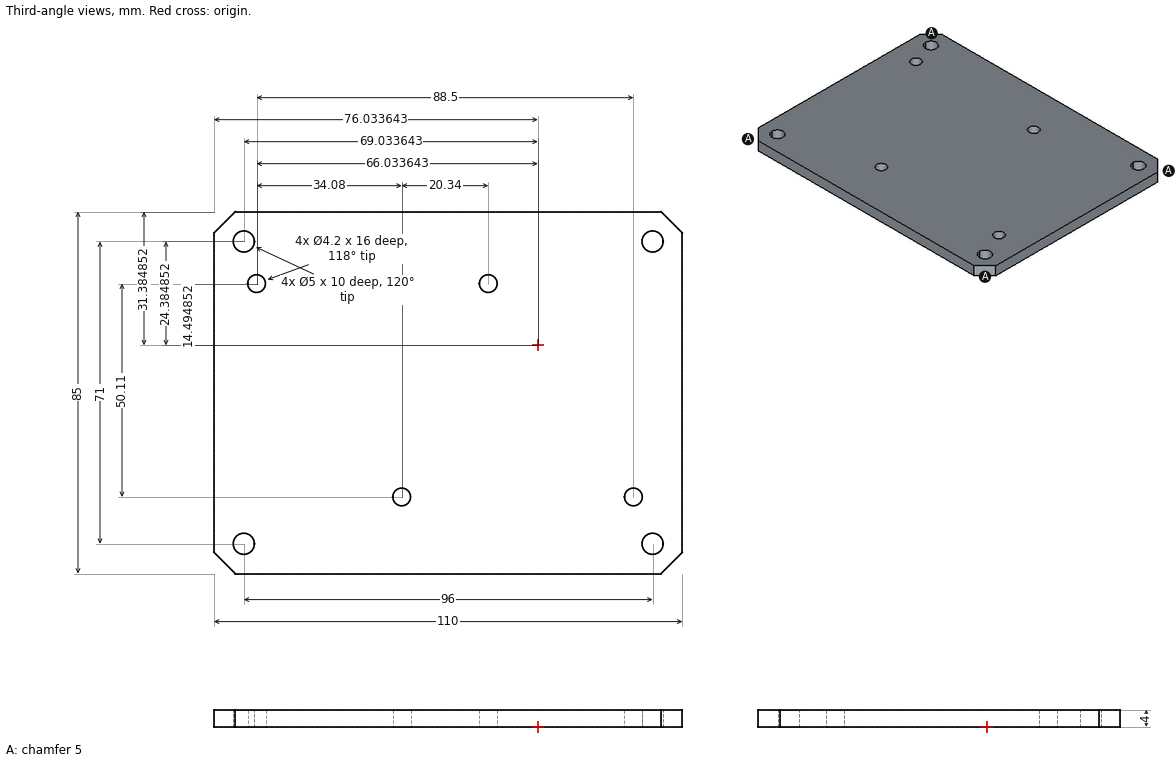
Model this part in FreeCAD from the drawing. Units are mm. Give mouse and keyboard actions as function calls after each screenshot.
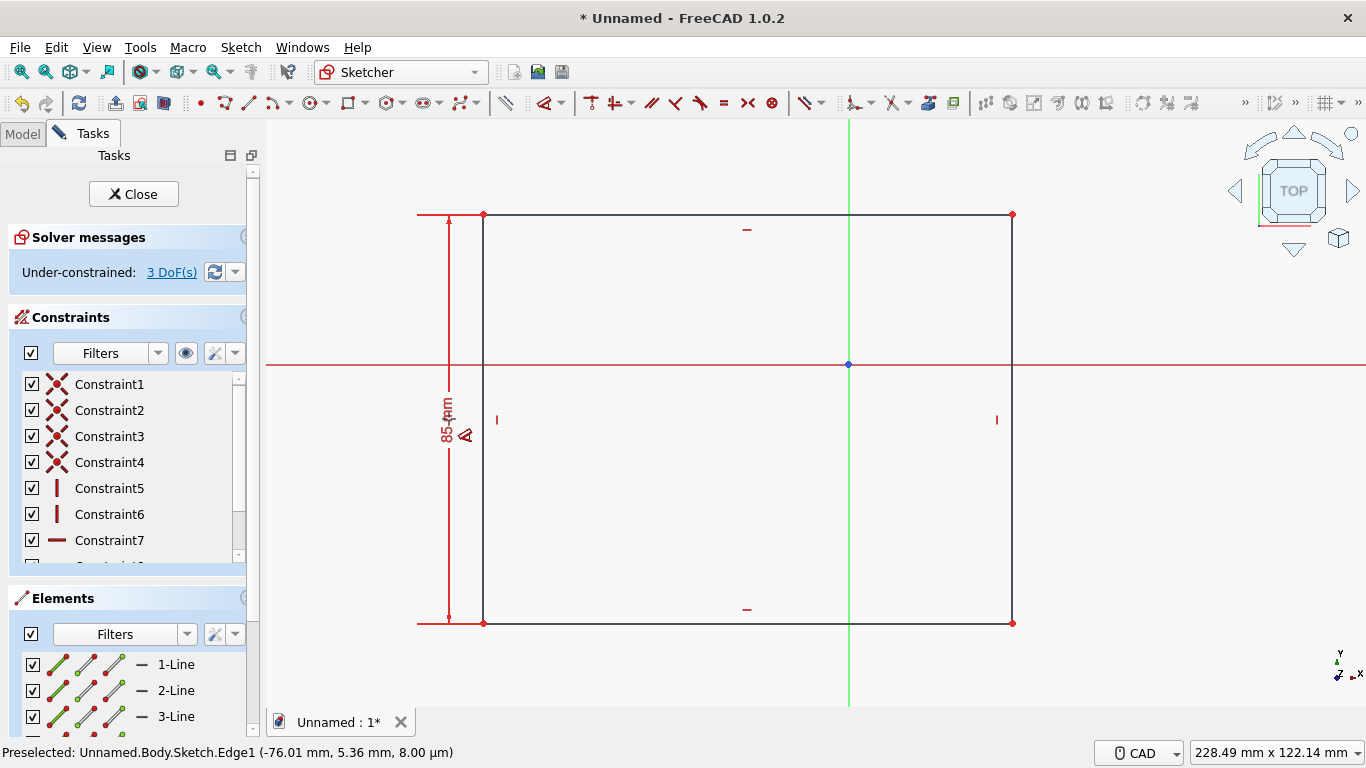
click(642, 624)
click(748, 658)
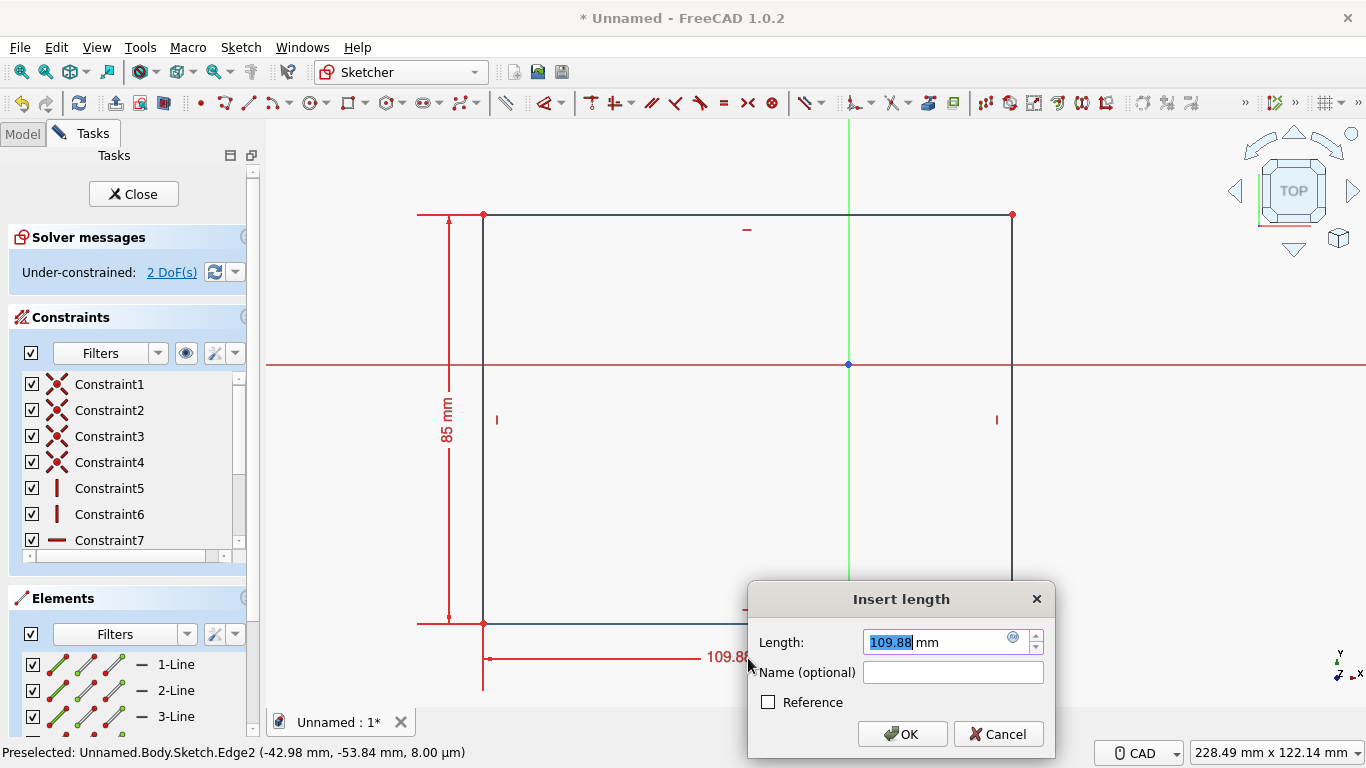
text(110)
key(Return)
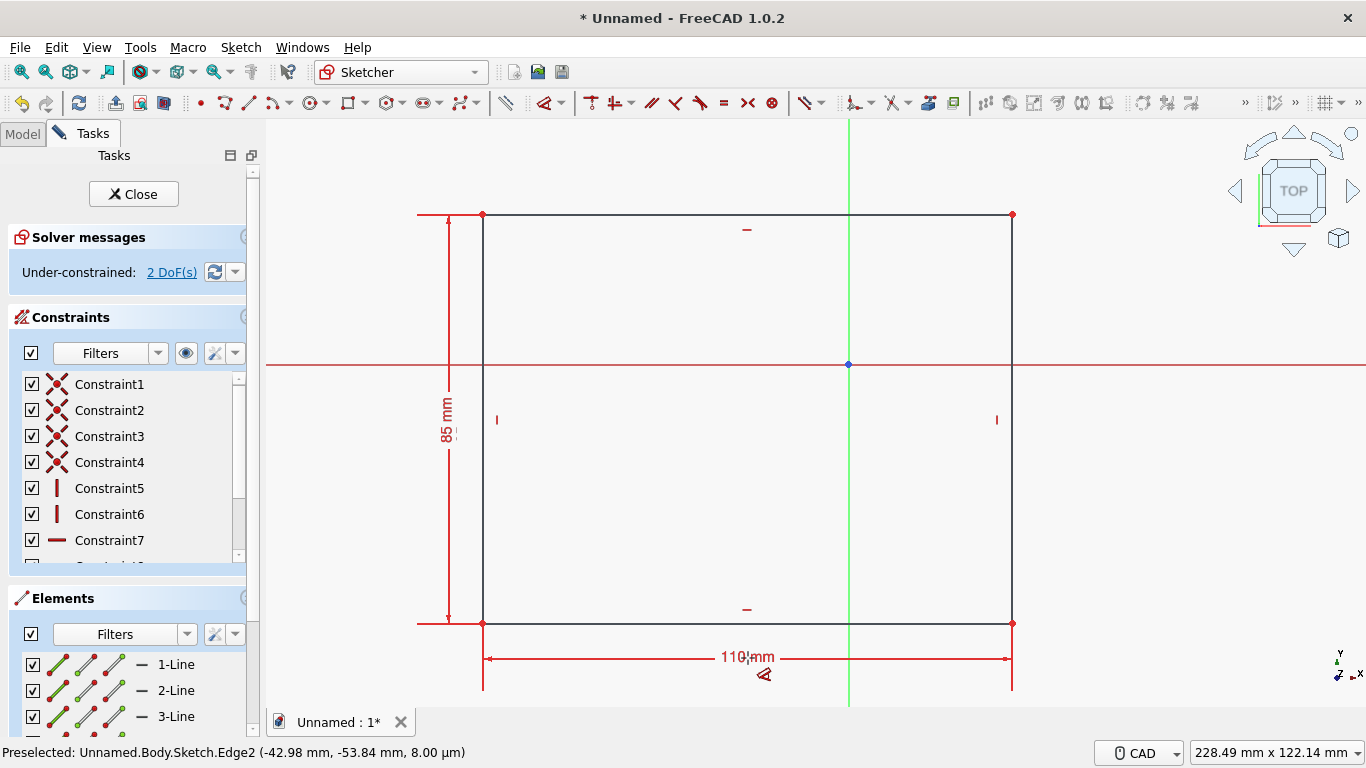
click(483, 215)
click(666, 181)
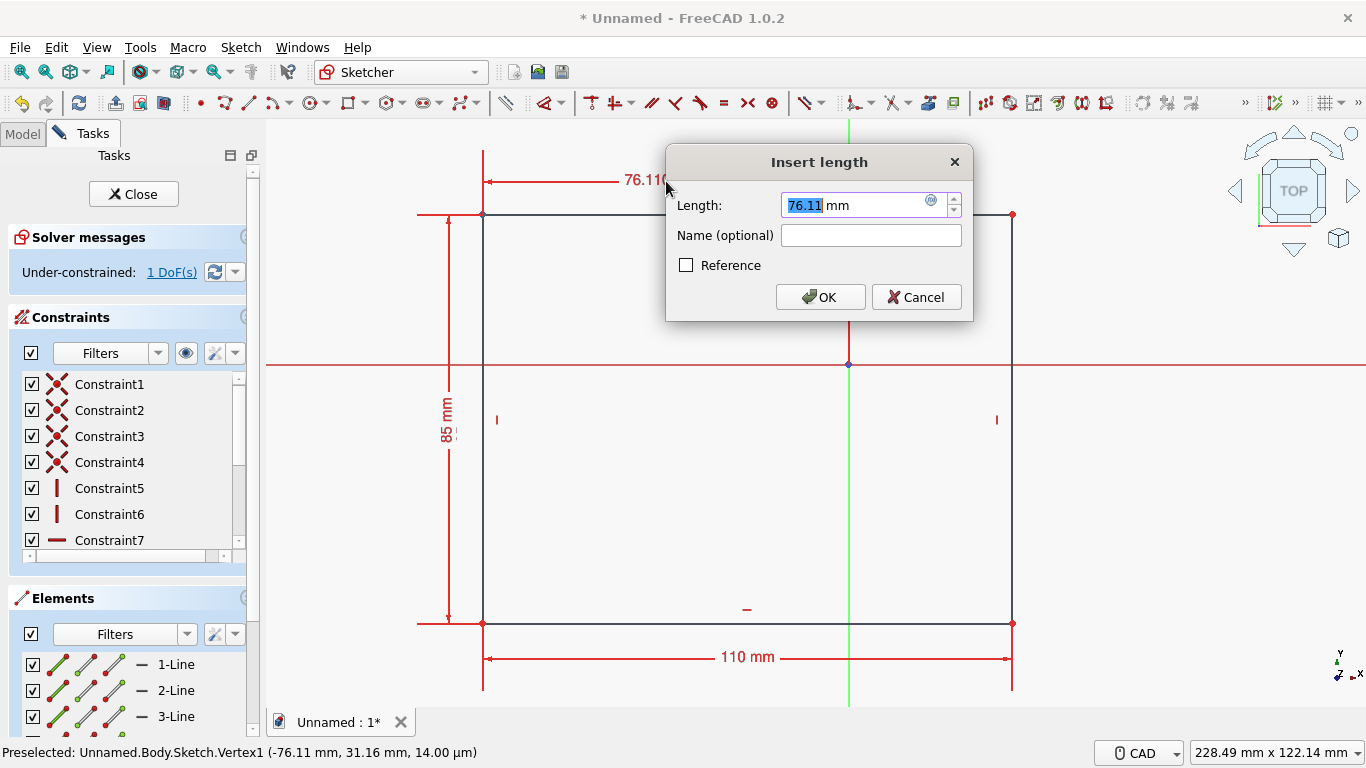
text(76.033643)
key(Return)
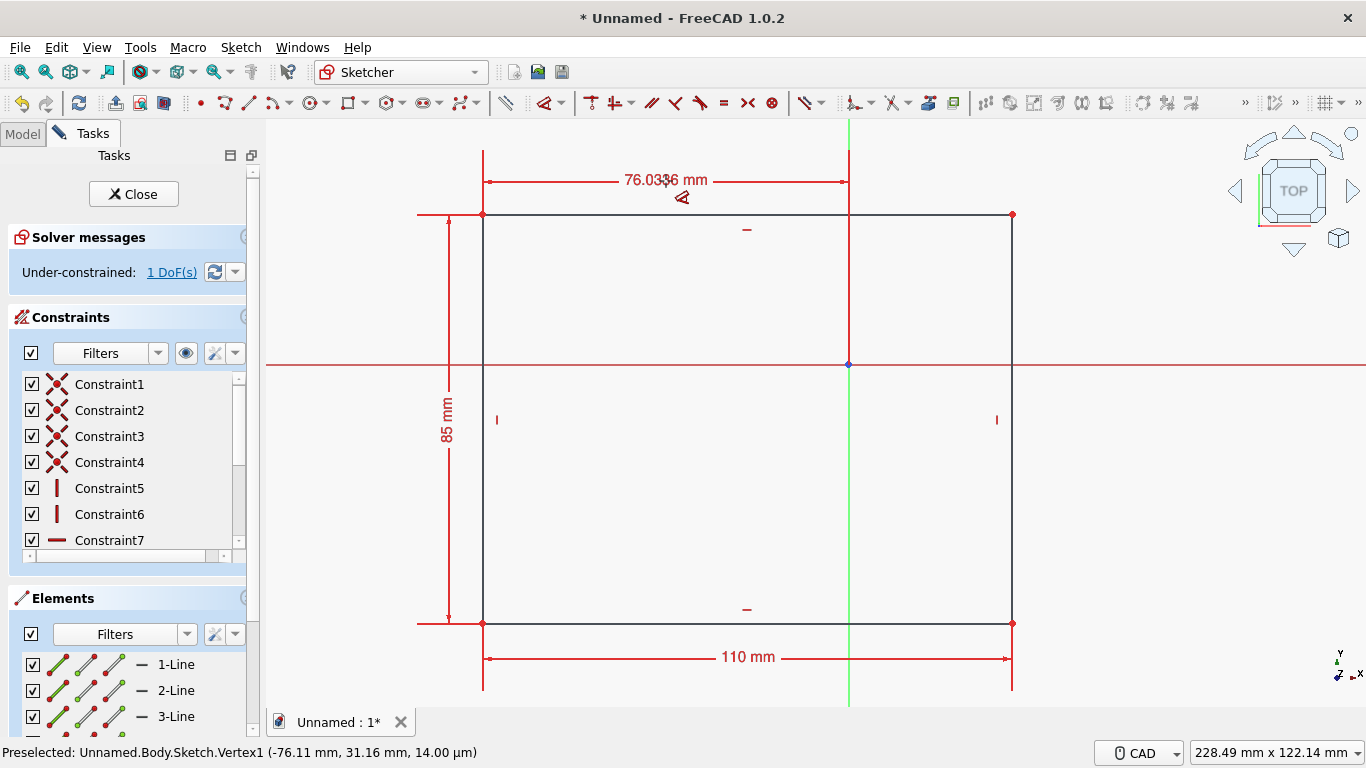
click(483, 215)
click(449, 290)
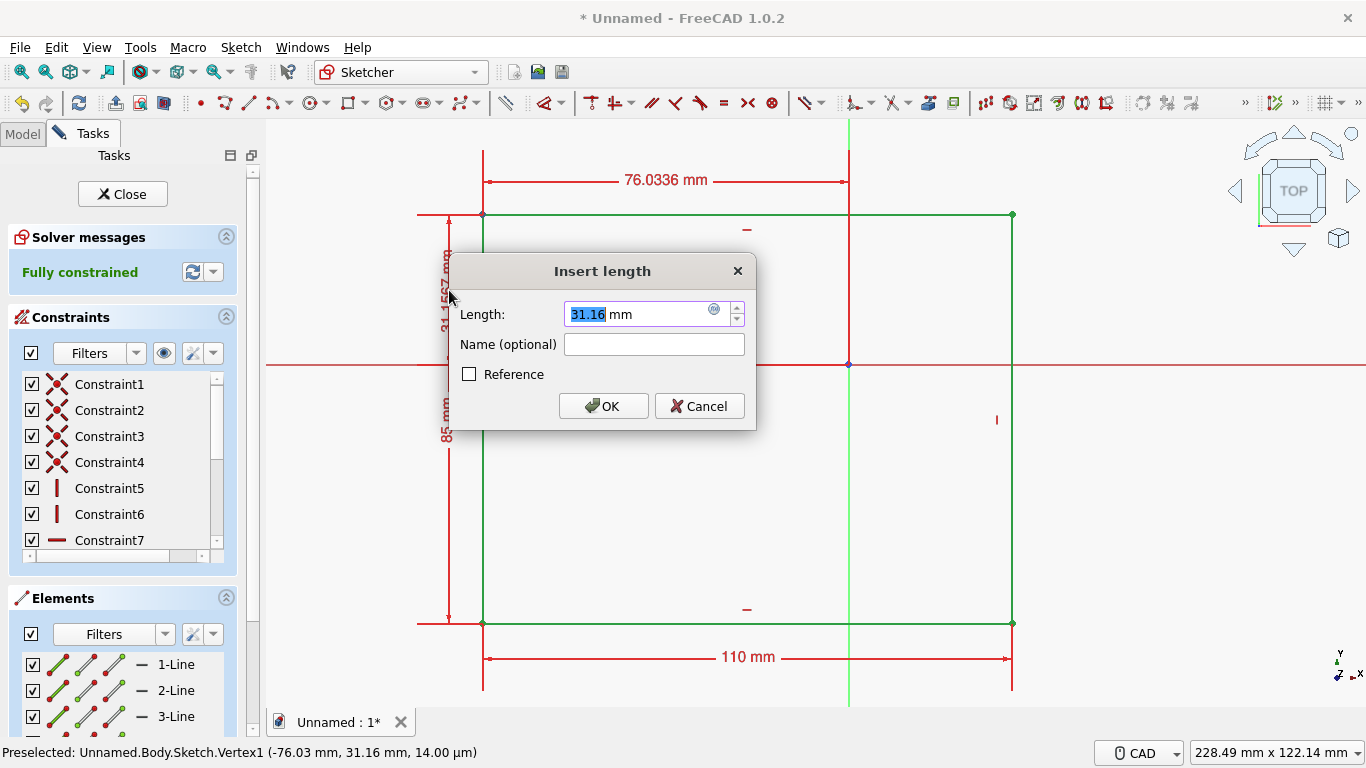
text(31.384852)
key(Return)
key(Escape)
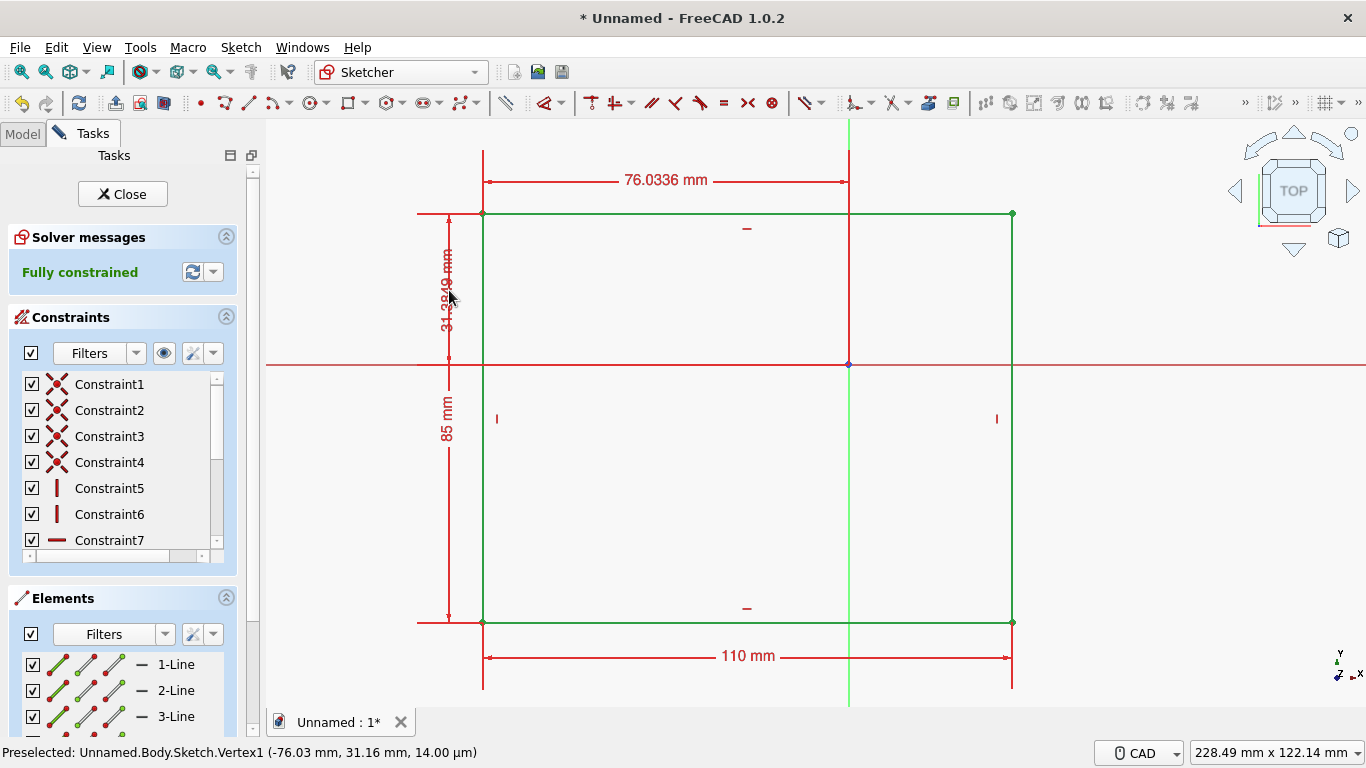
click(123, 194)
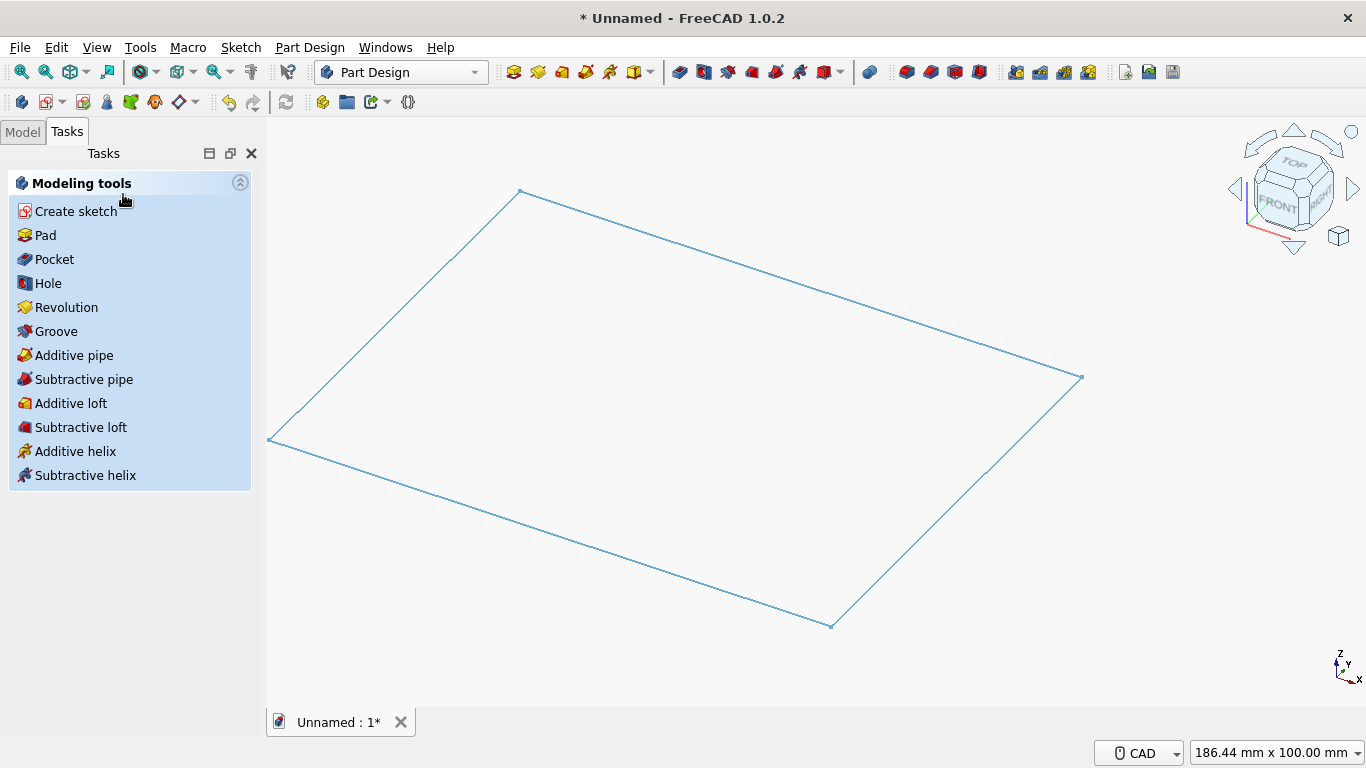
click(514, 72)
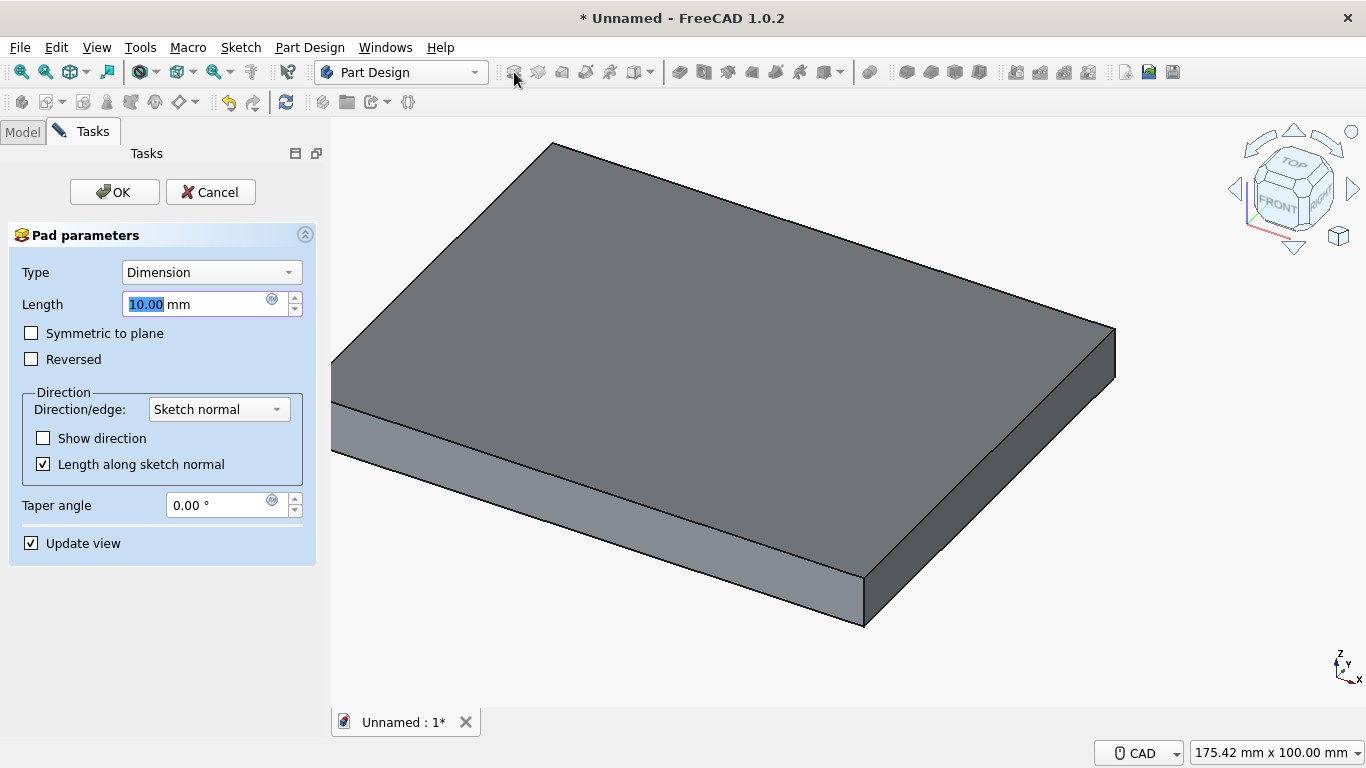
text(4)
key(Tab)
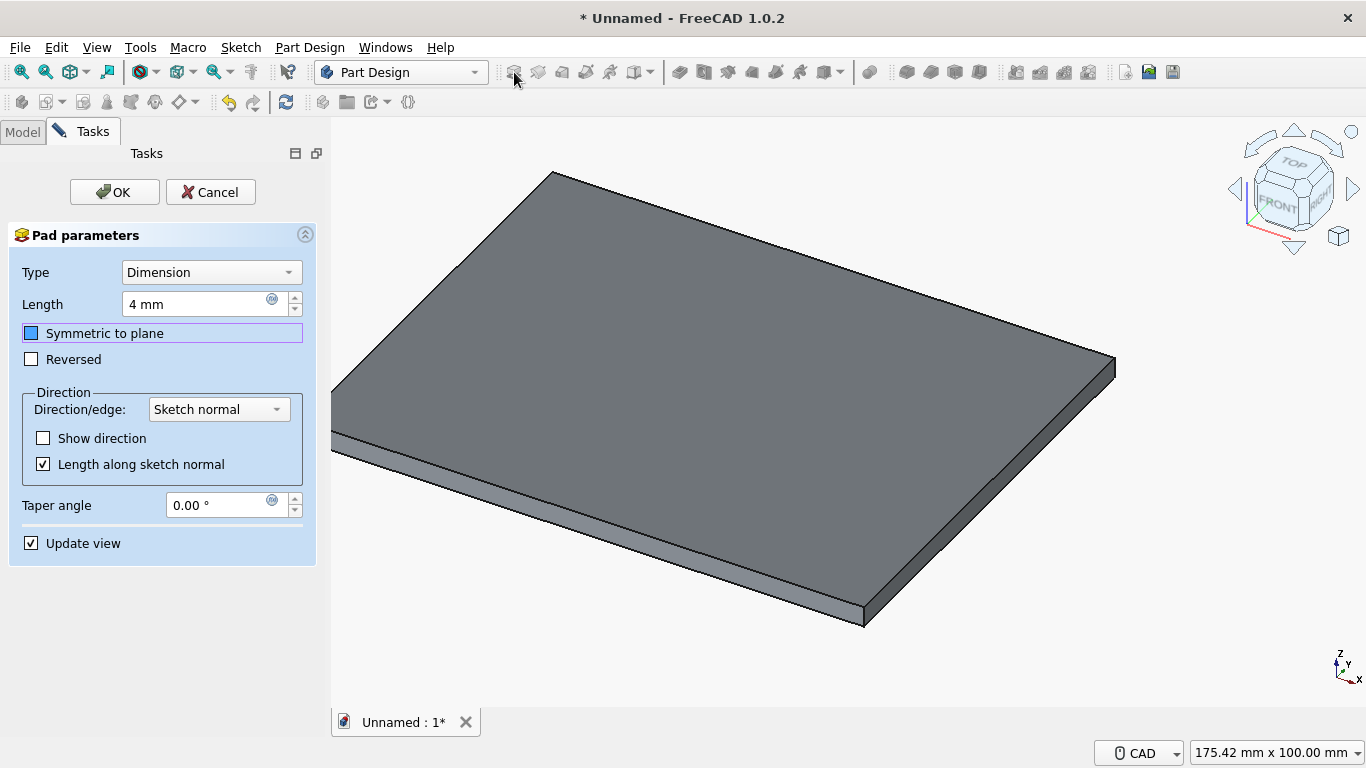
click(115, 192)